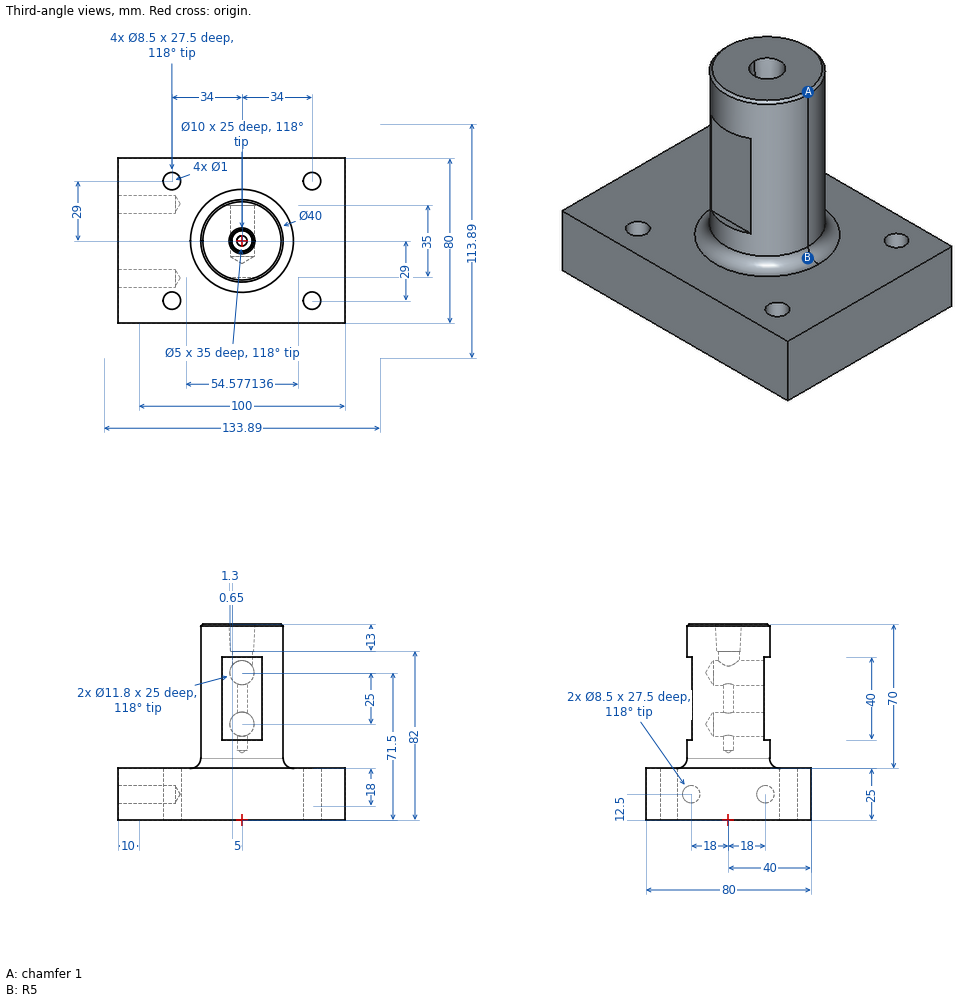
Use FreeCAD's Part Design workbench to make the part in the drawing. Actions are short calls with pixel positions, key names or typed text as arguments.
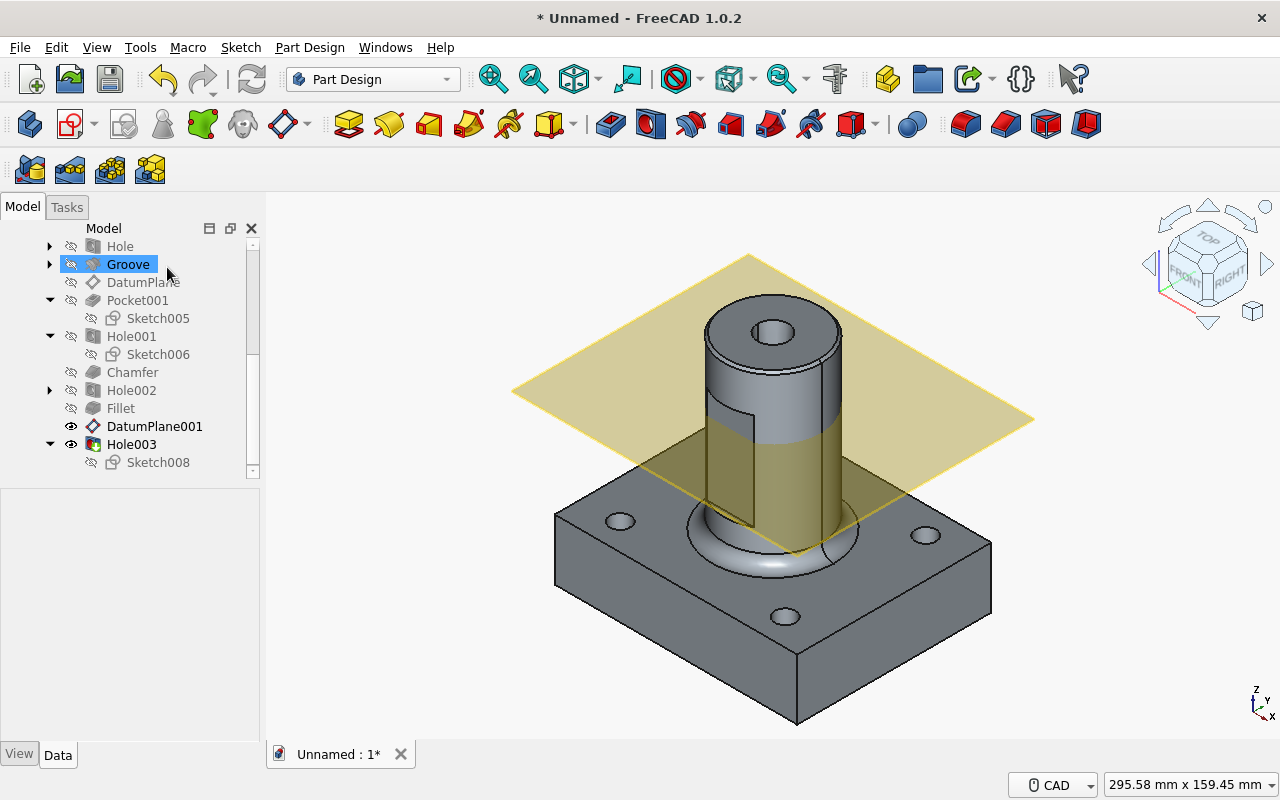
click(116, 426)
key(space)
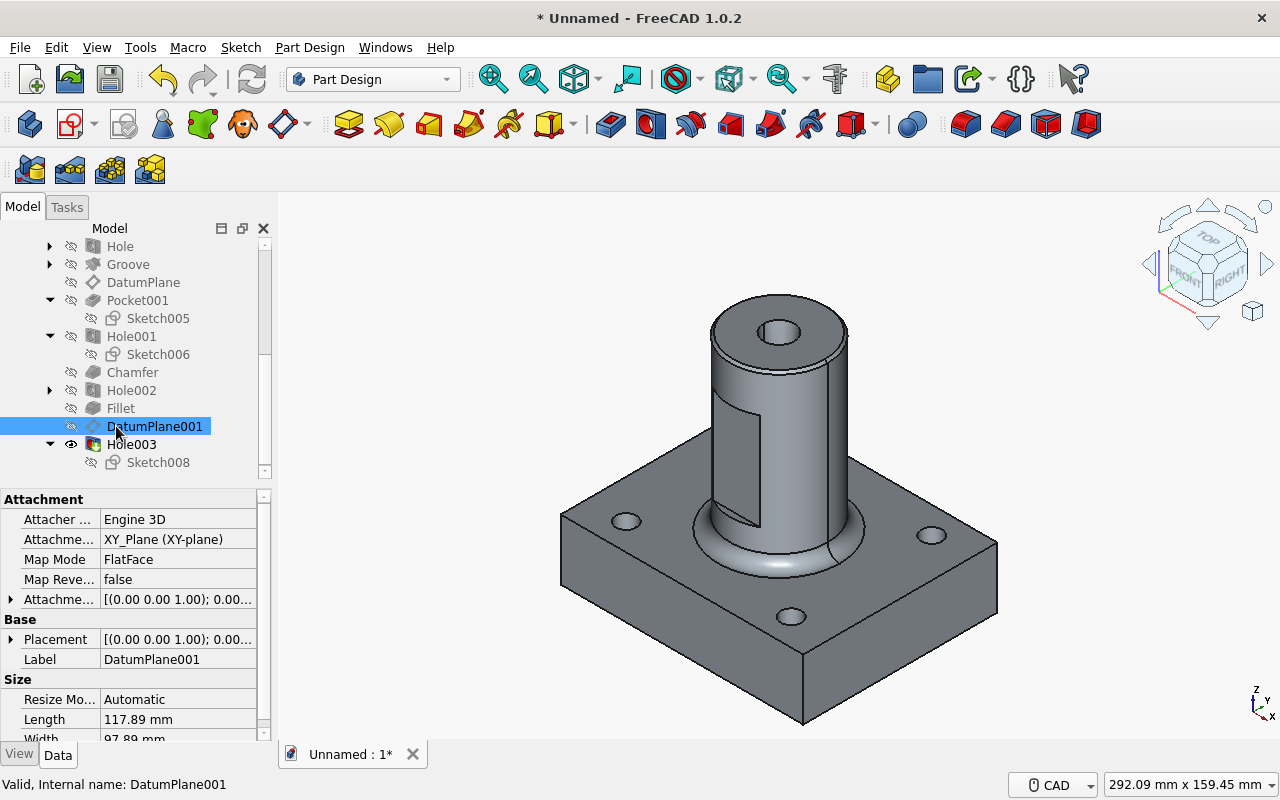
key(6)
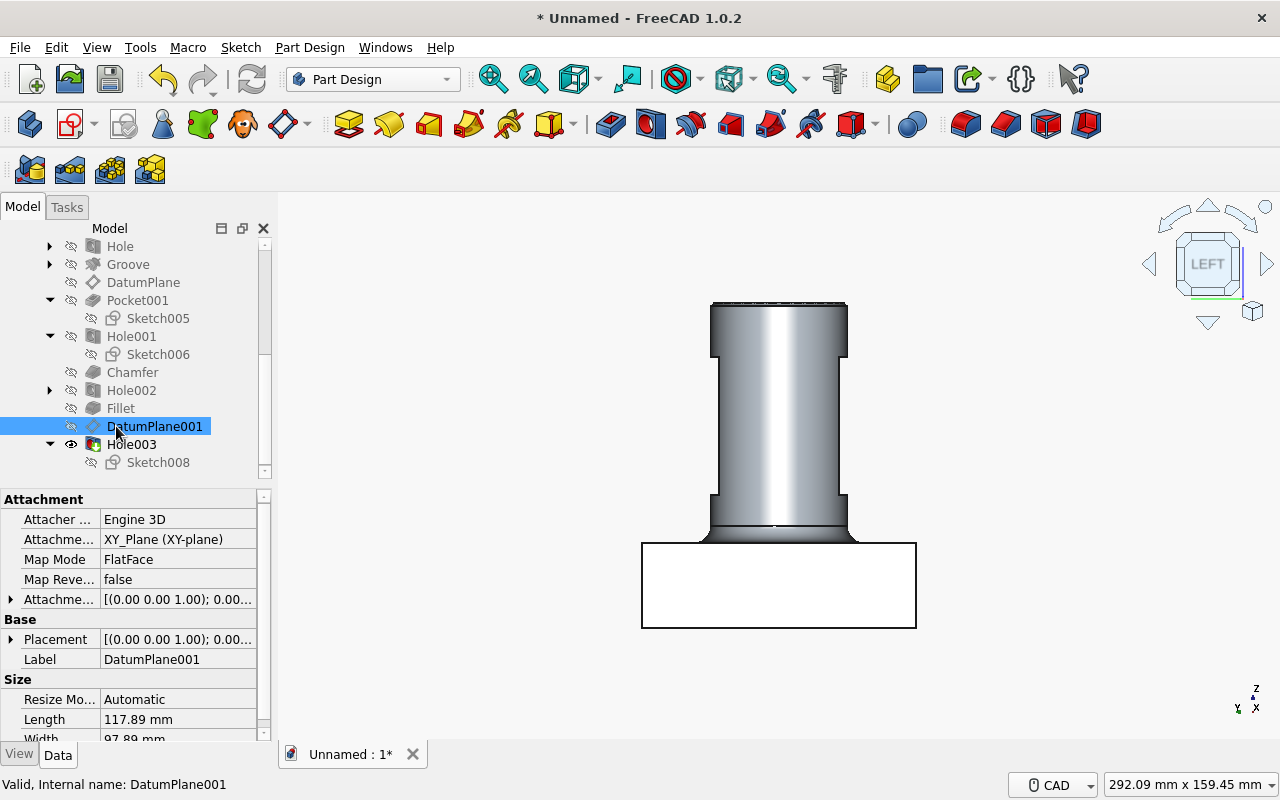
click(701, 585)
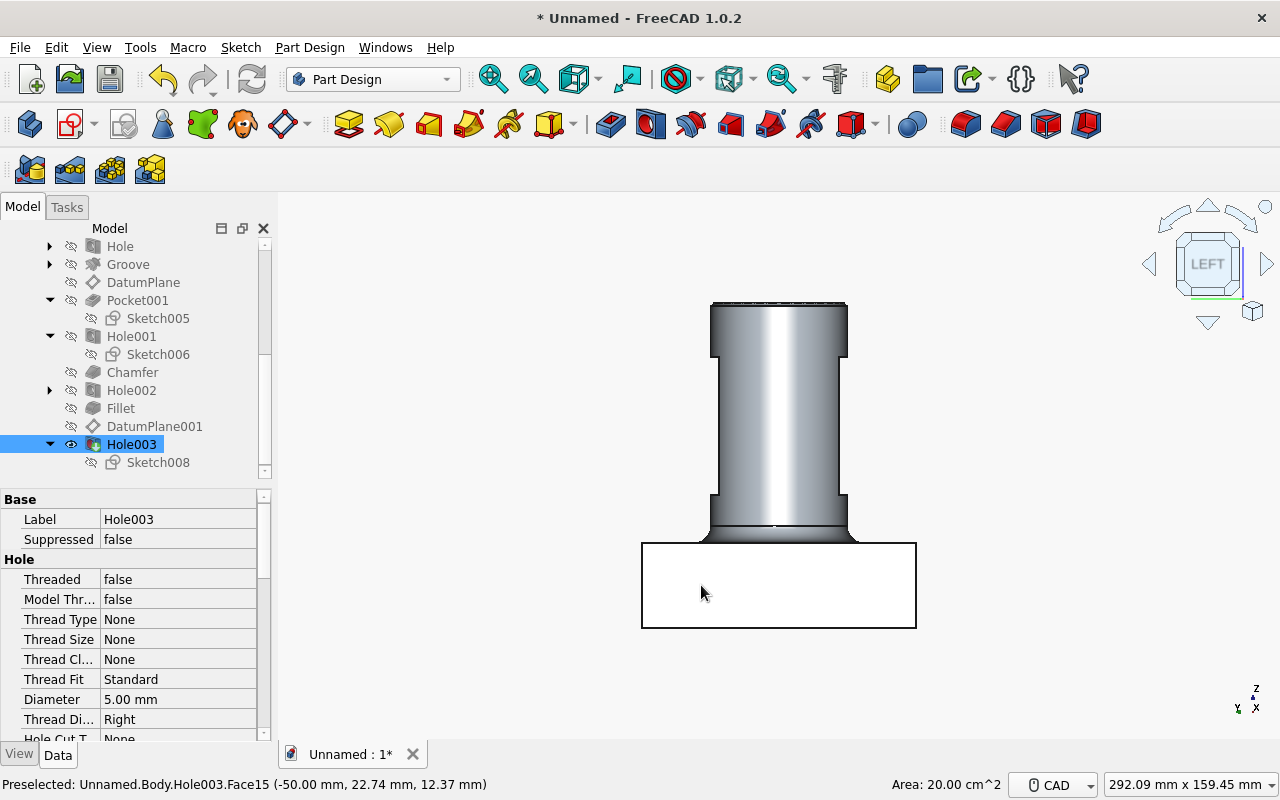
click(70, 124)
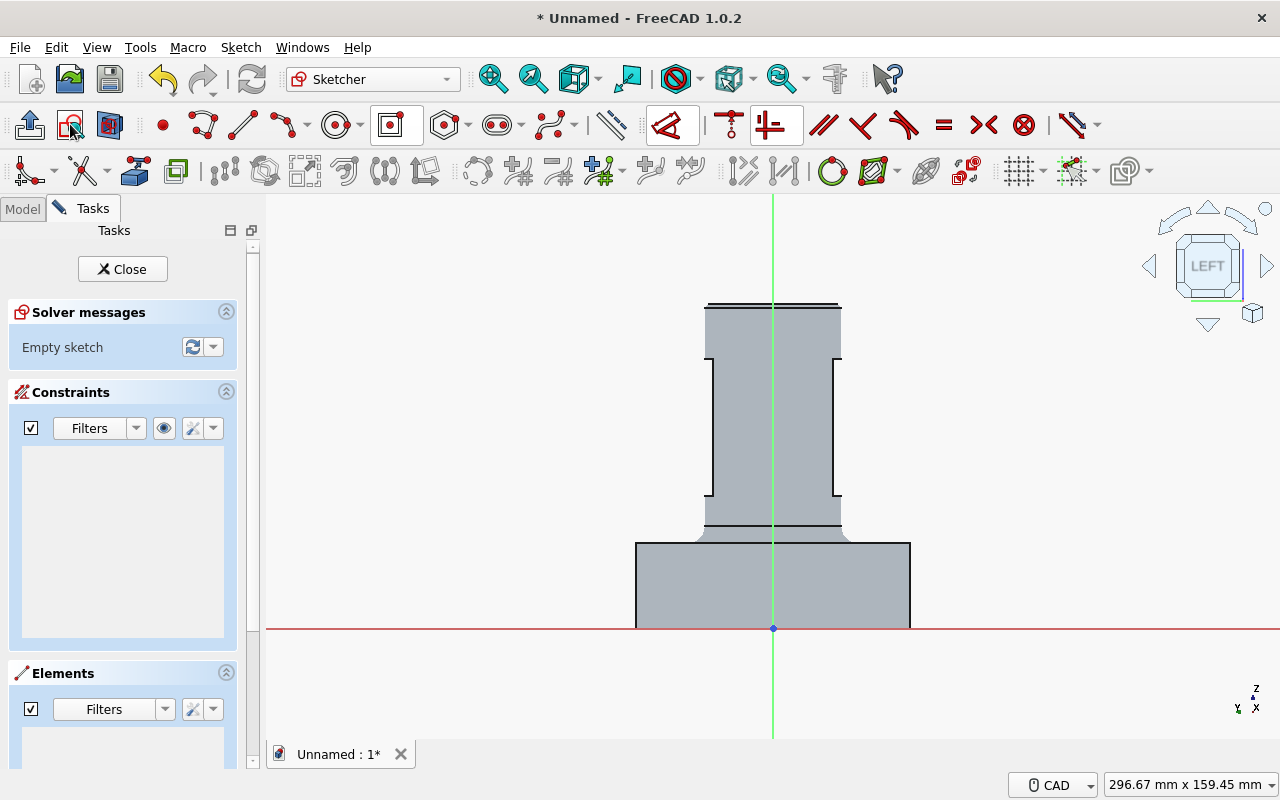
scroll(829, 684, up, 4)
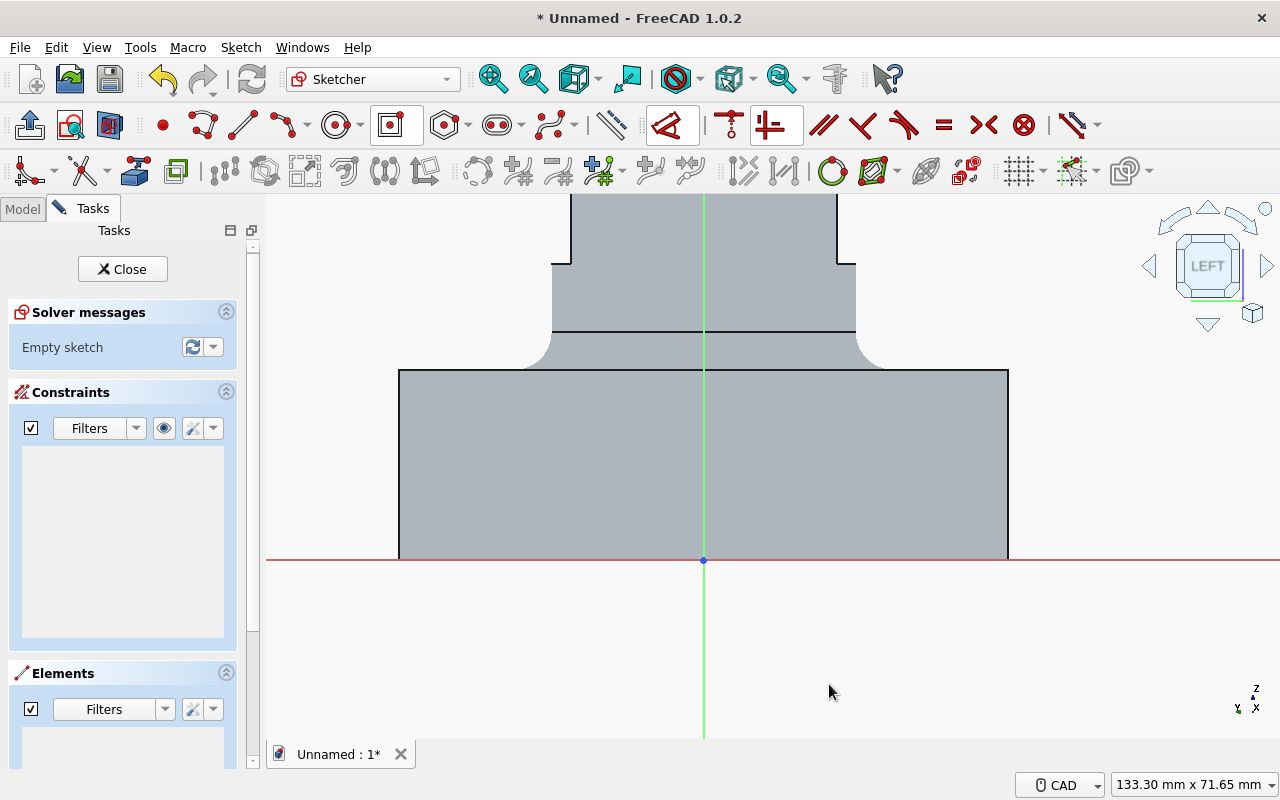
key(g)
key(r)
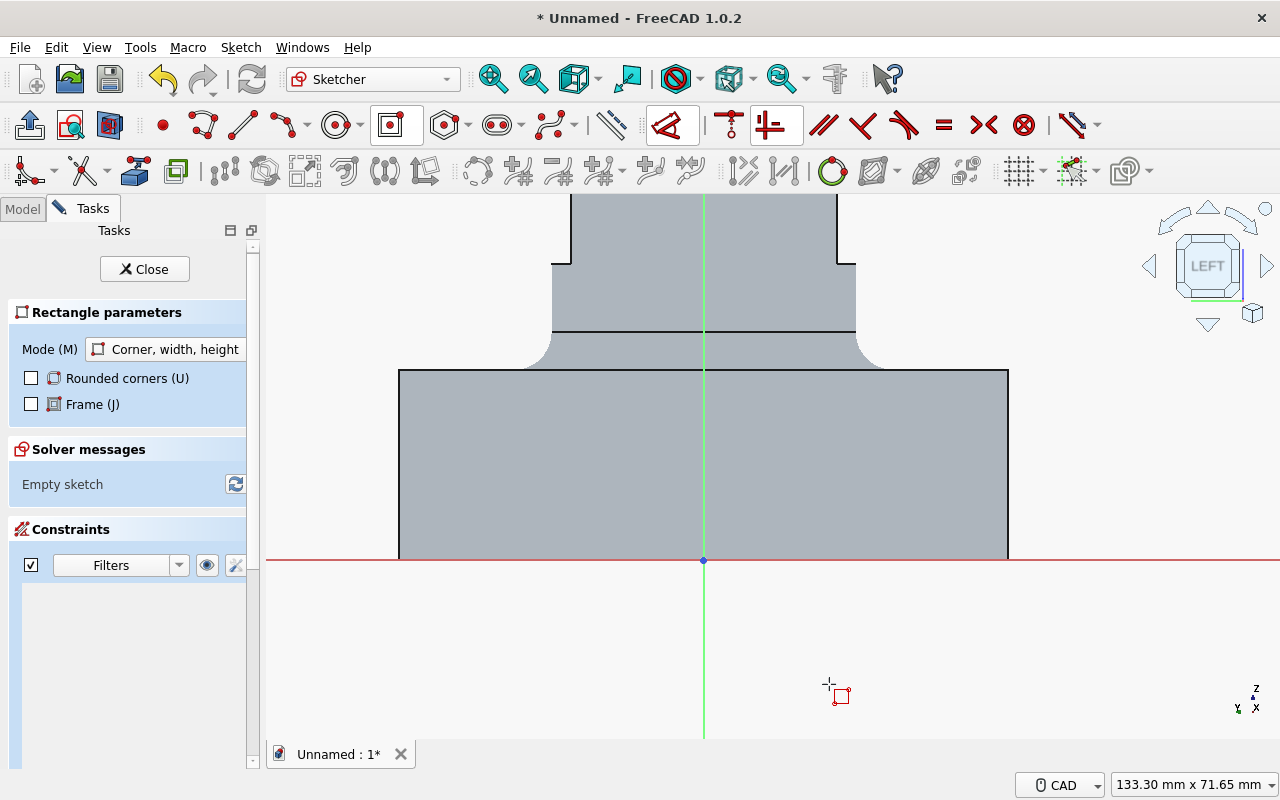
click(399, 370)
click(1008, 560)
key(Escape)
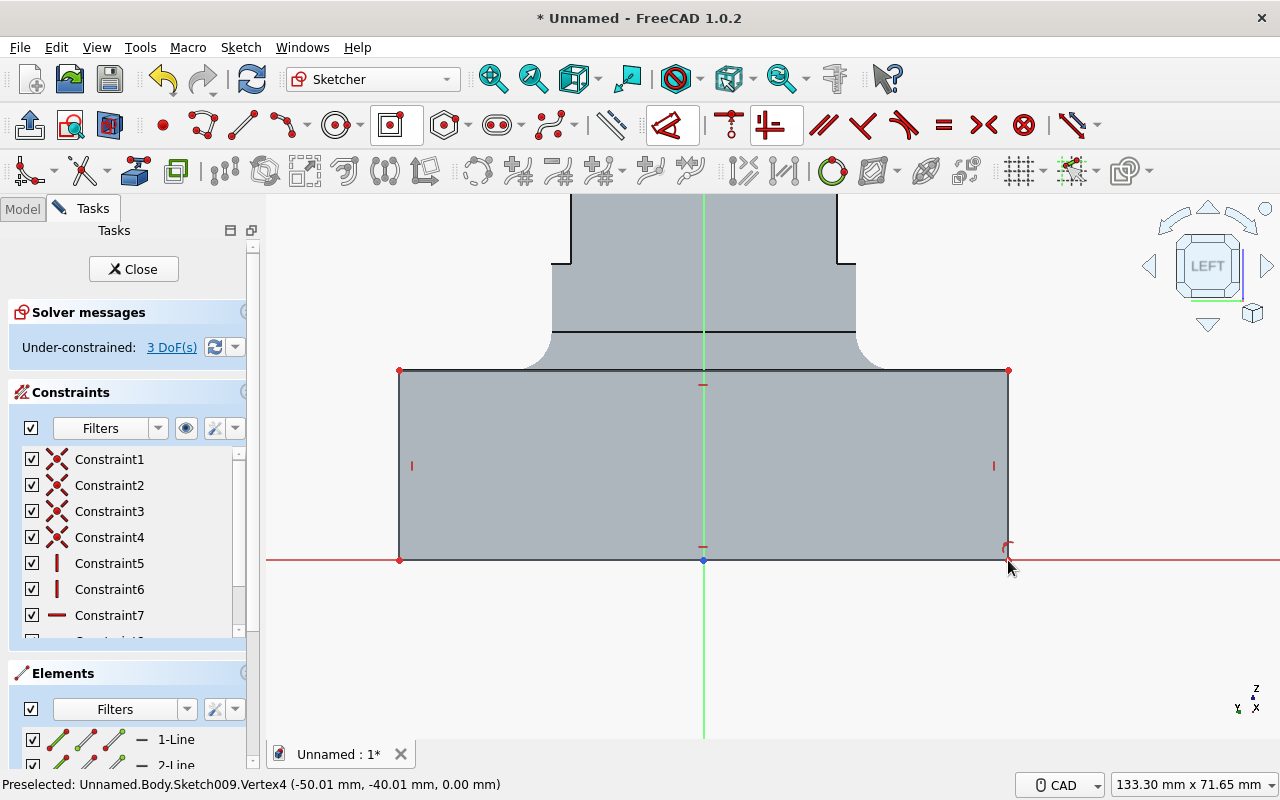
click(399, 428)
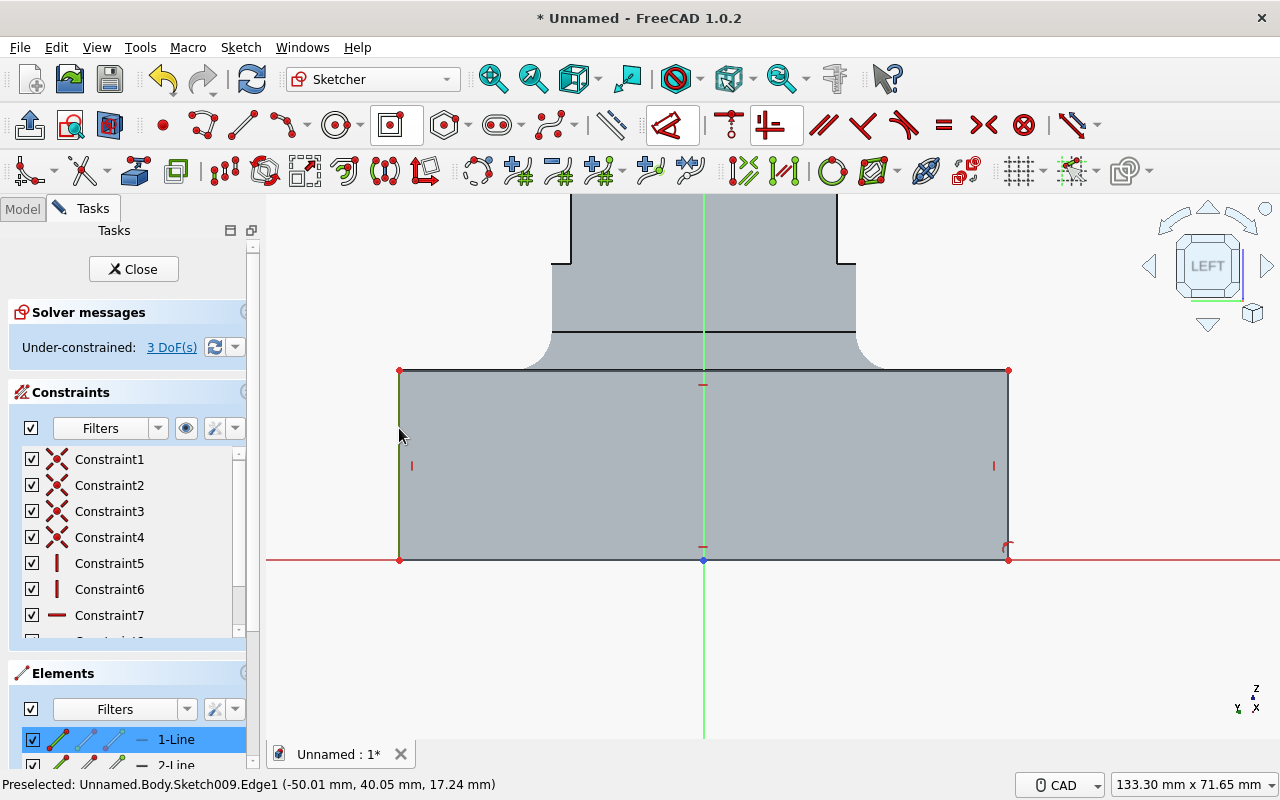
key(i)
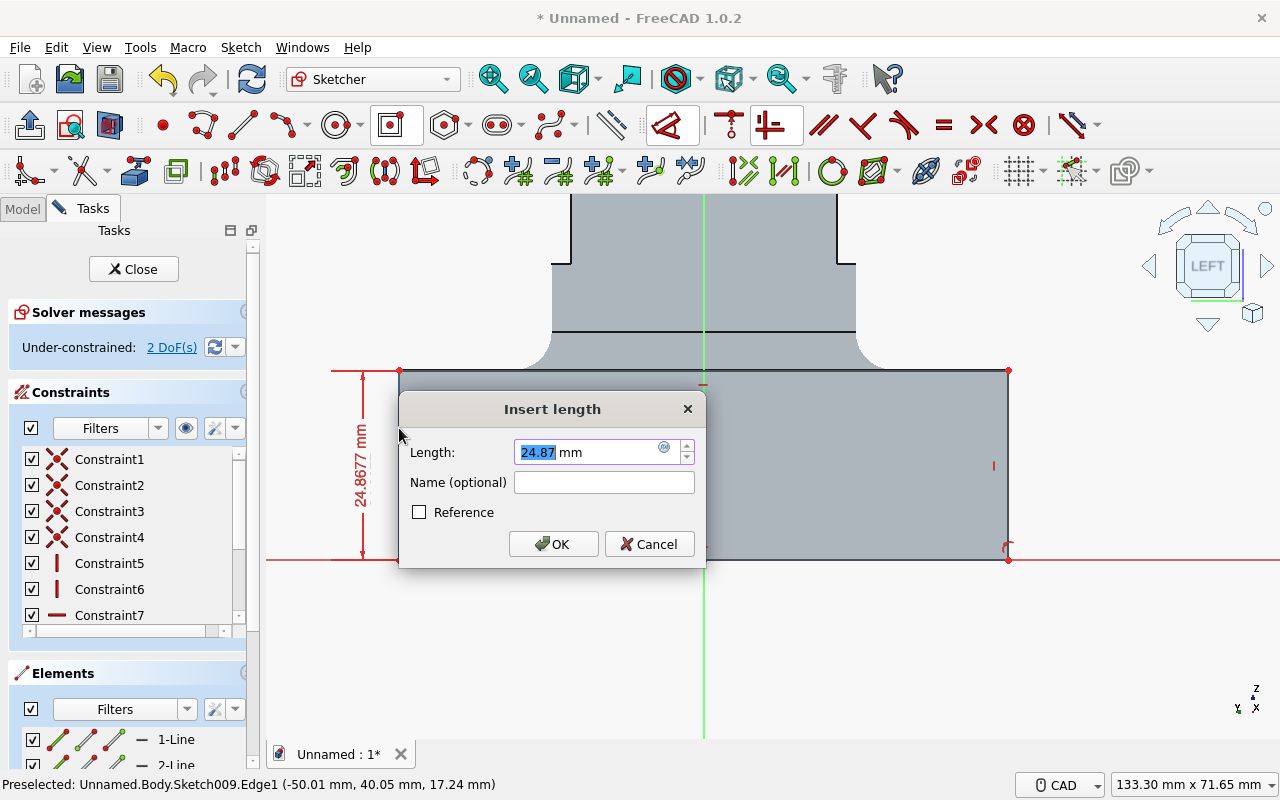
text(25)
key(Return)